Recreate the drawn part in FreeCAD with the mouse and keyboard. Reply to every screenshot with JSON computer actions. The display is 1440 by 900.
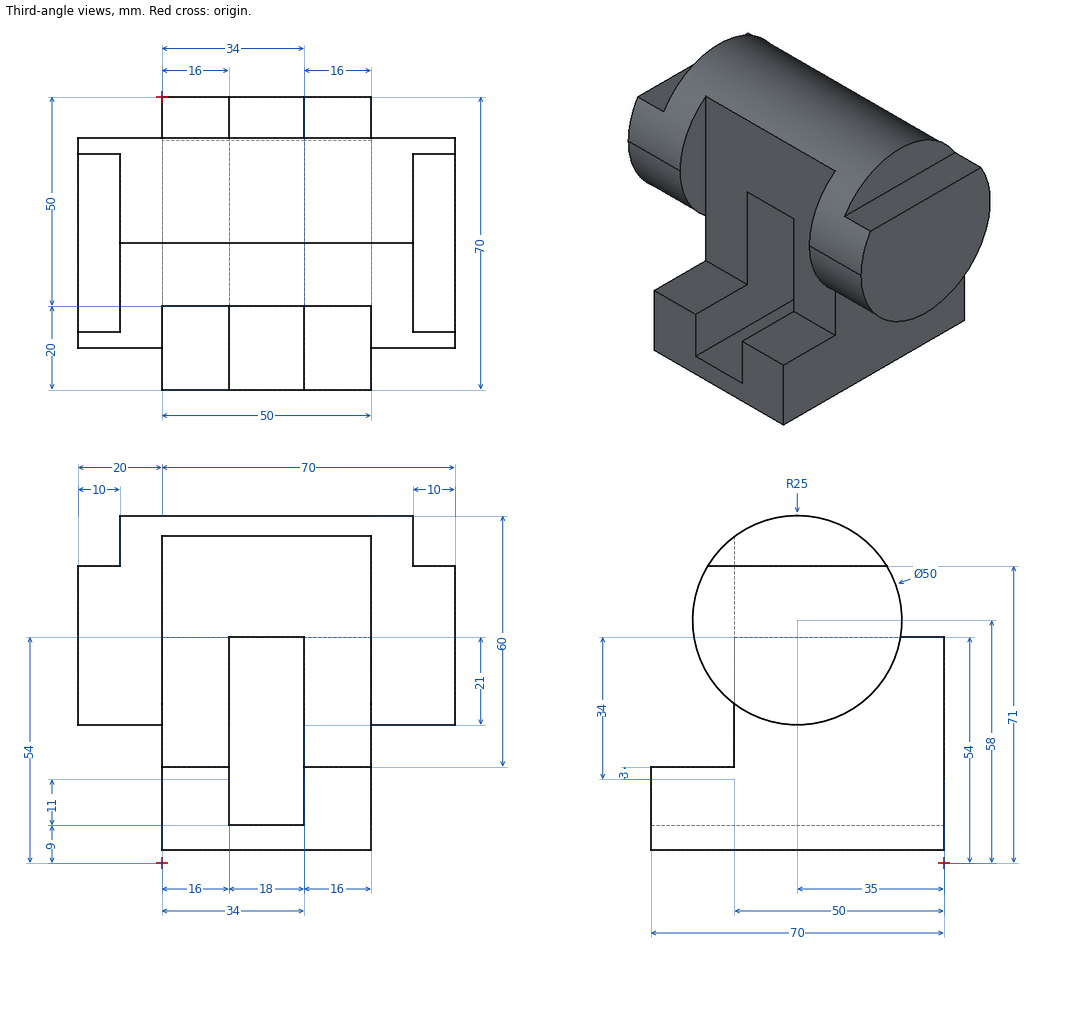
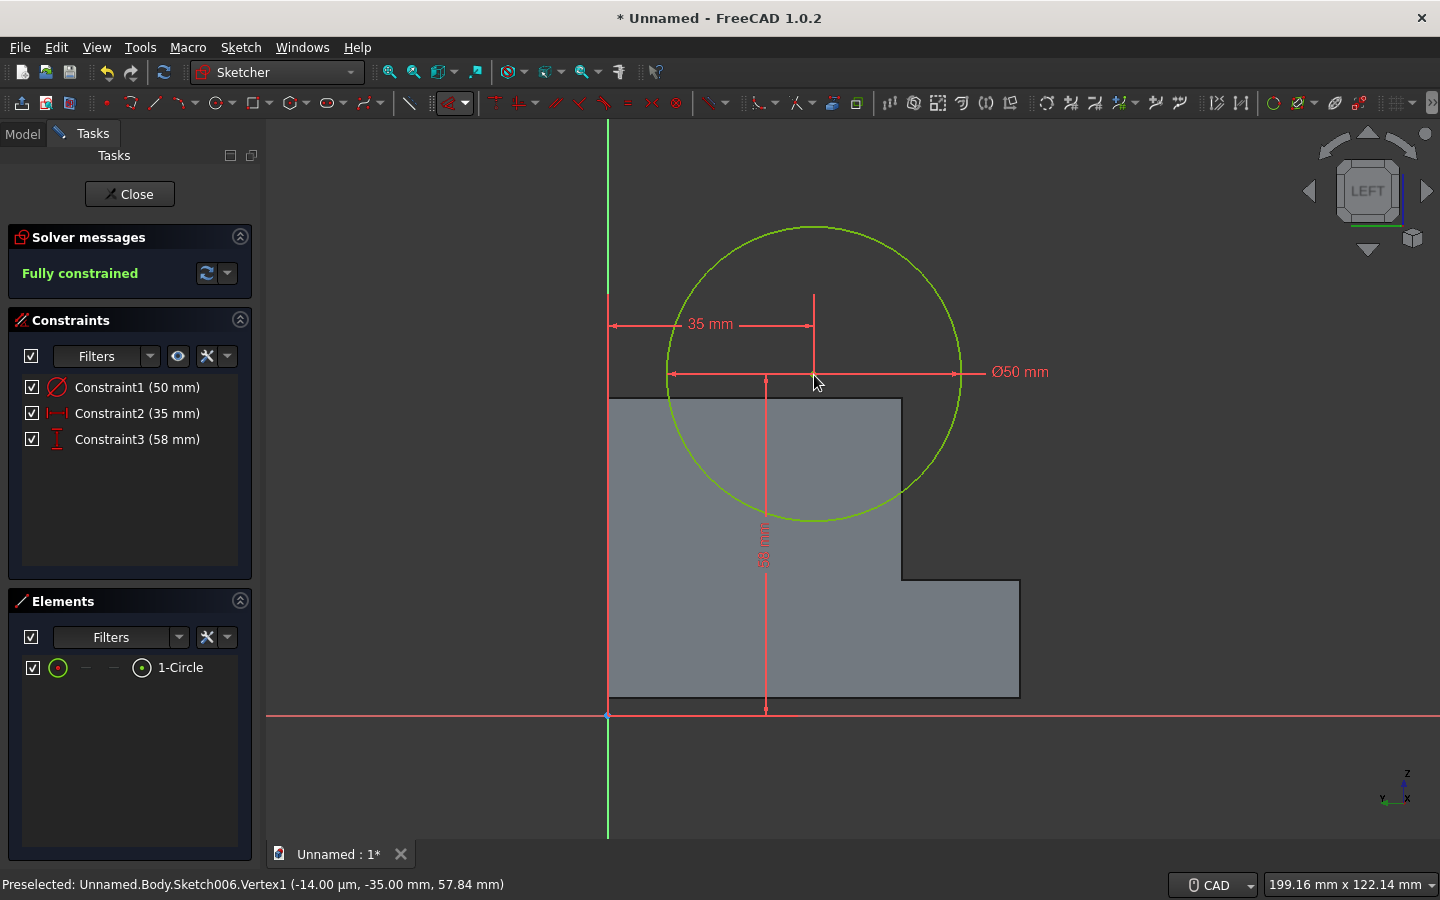
{"action": "left_click", "coordinate": [130, 194]}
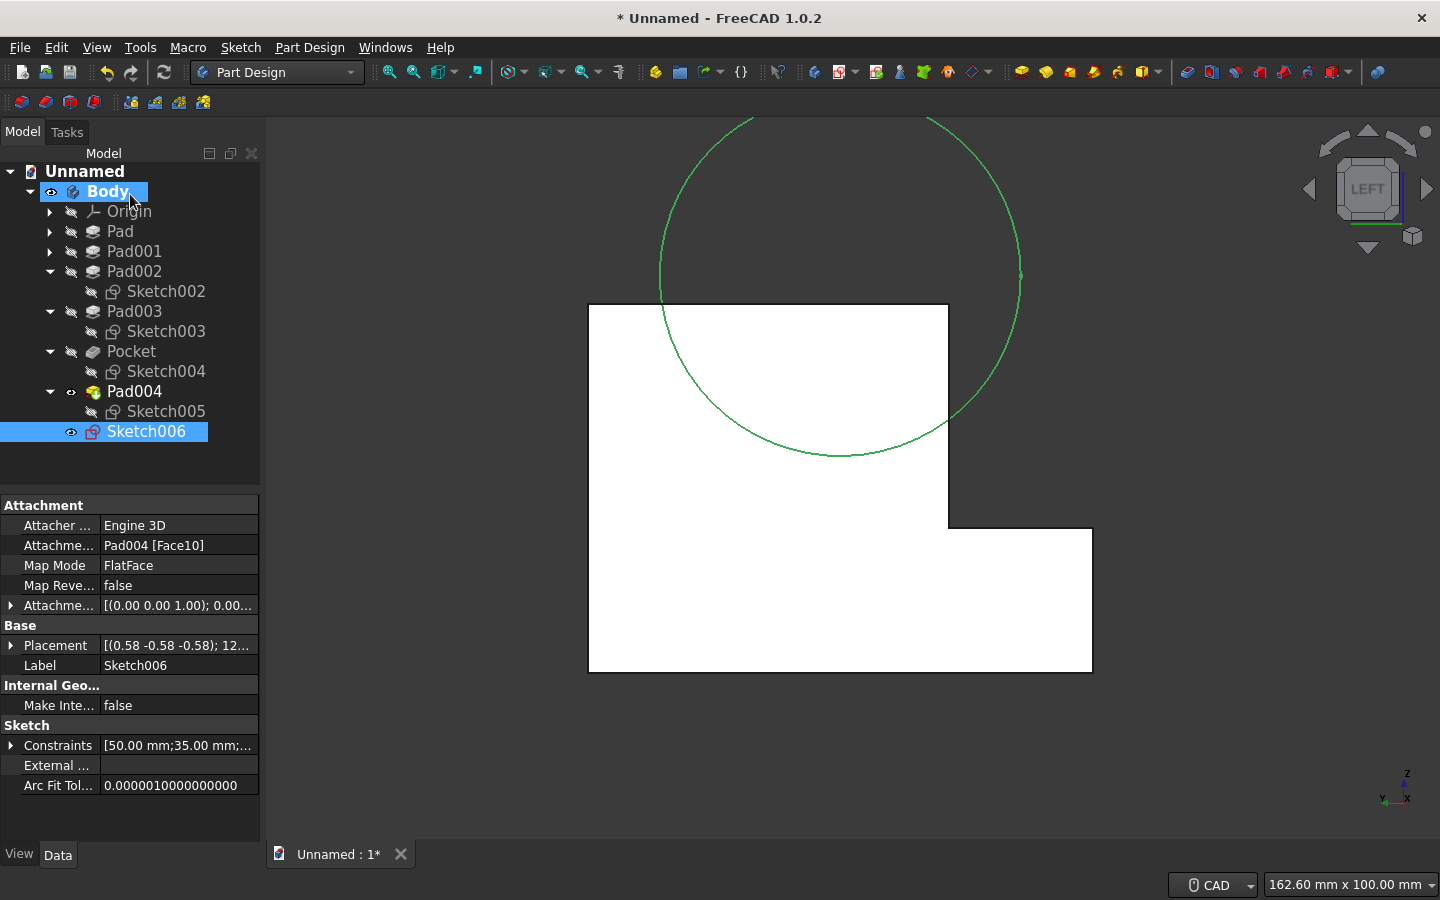
{"action": "left_click", "coordinate": [1022, 72]}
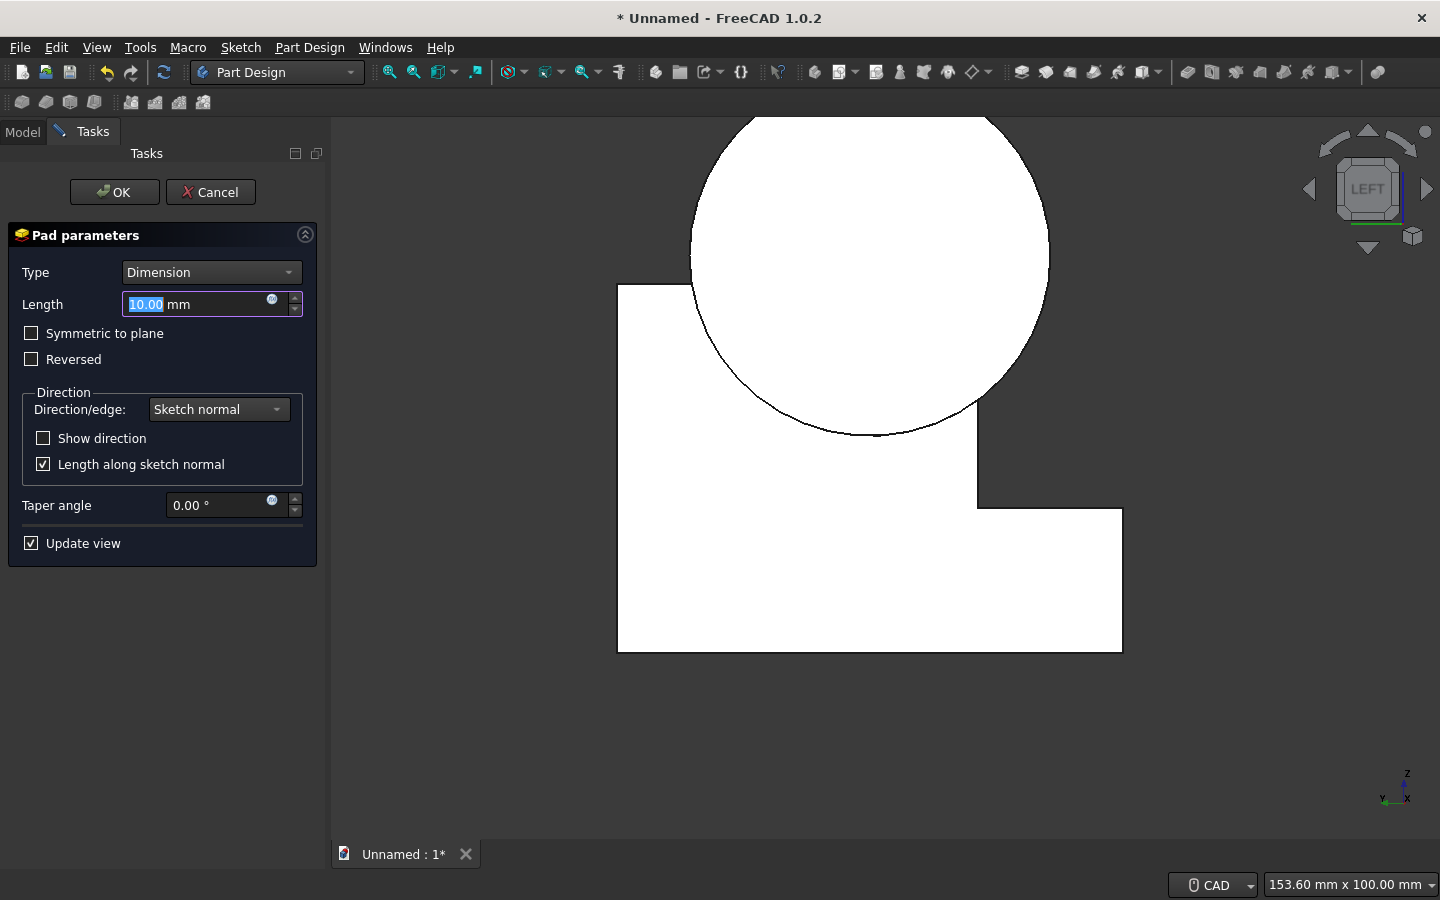
{"action": "type", "text": "70"}
{"action": "key", "text": "Tab"}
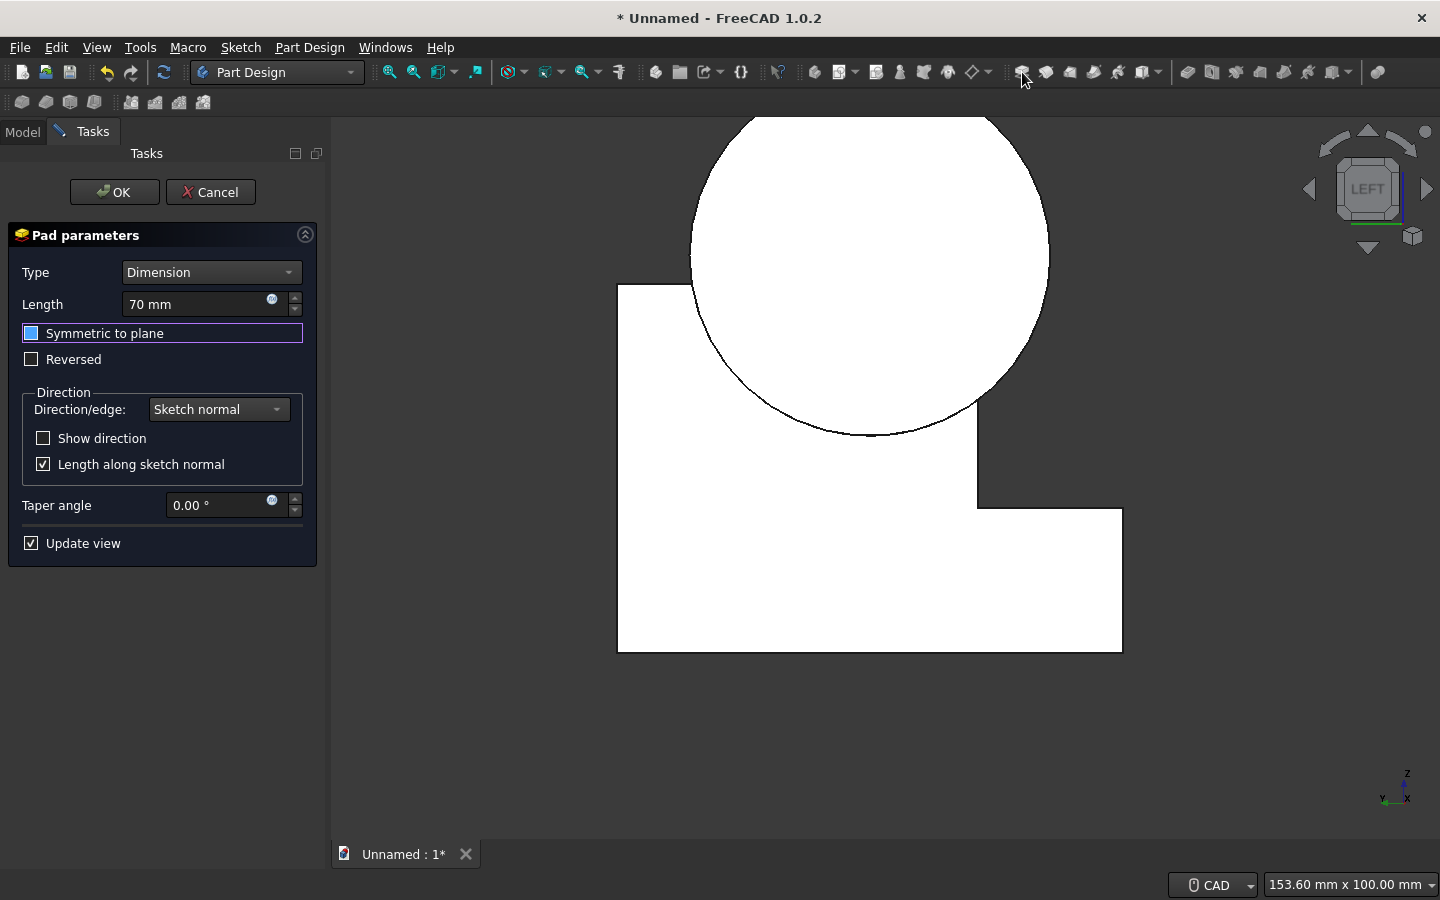
{"action": "left_click", "coordinate": [30, 359]}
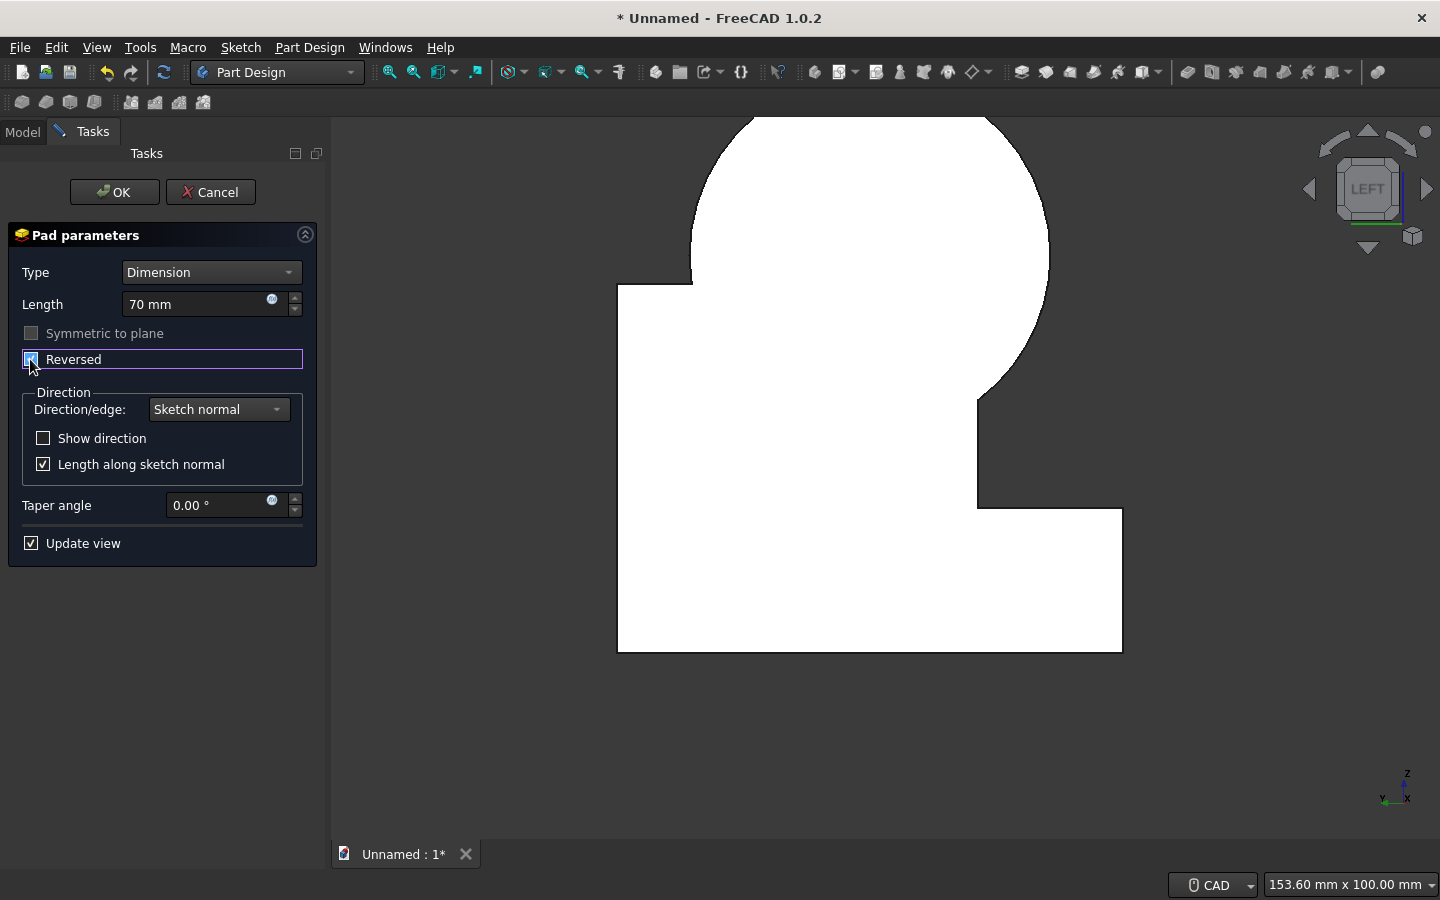
{"action": "left_click", "coordinate": [115, 192]}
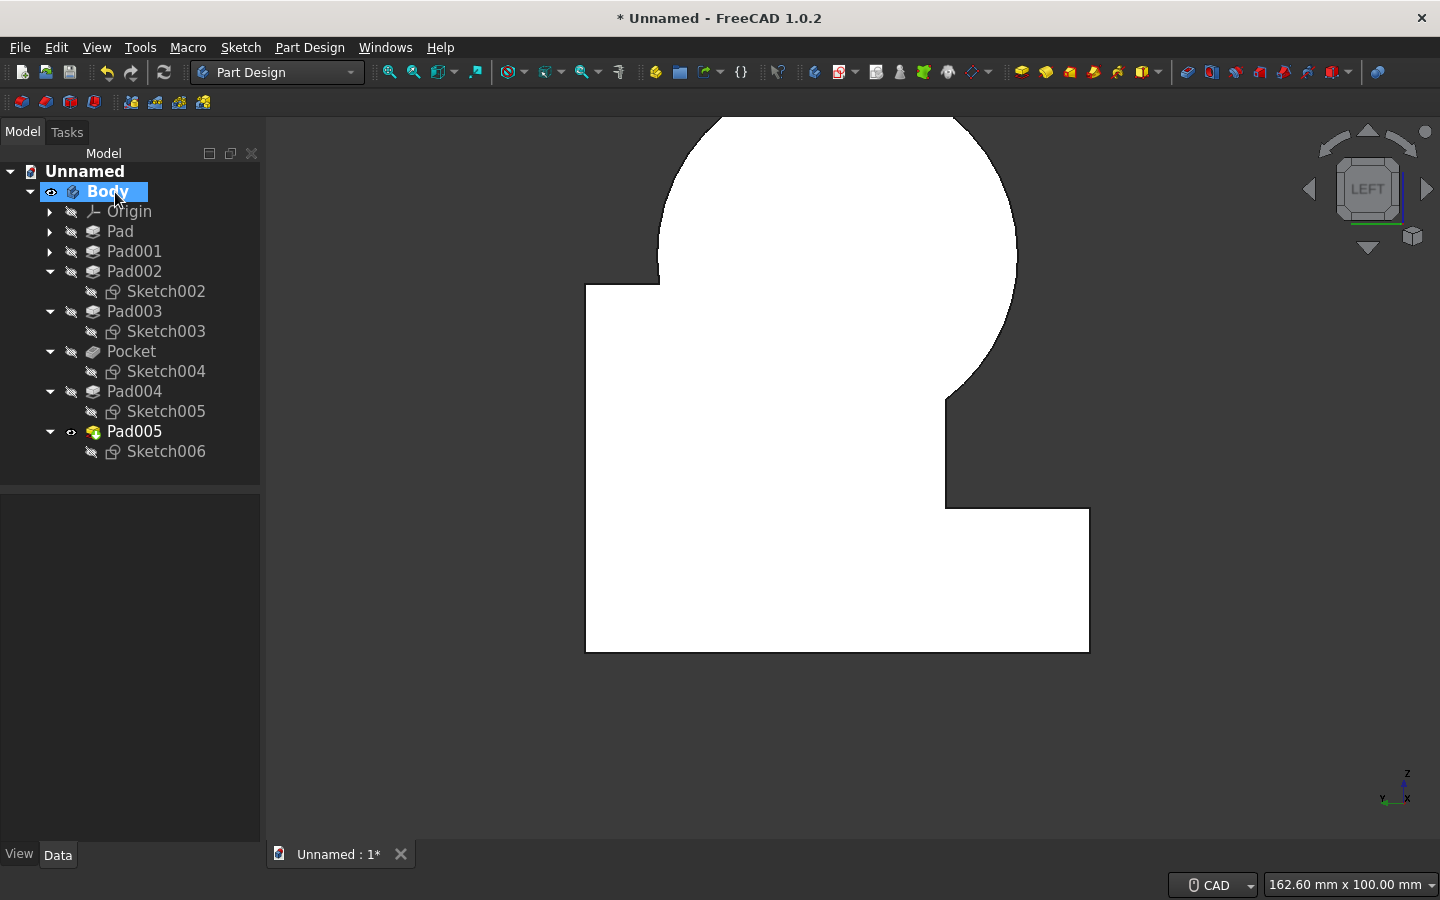
{"action": "key", "text": "v f"}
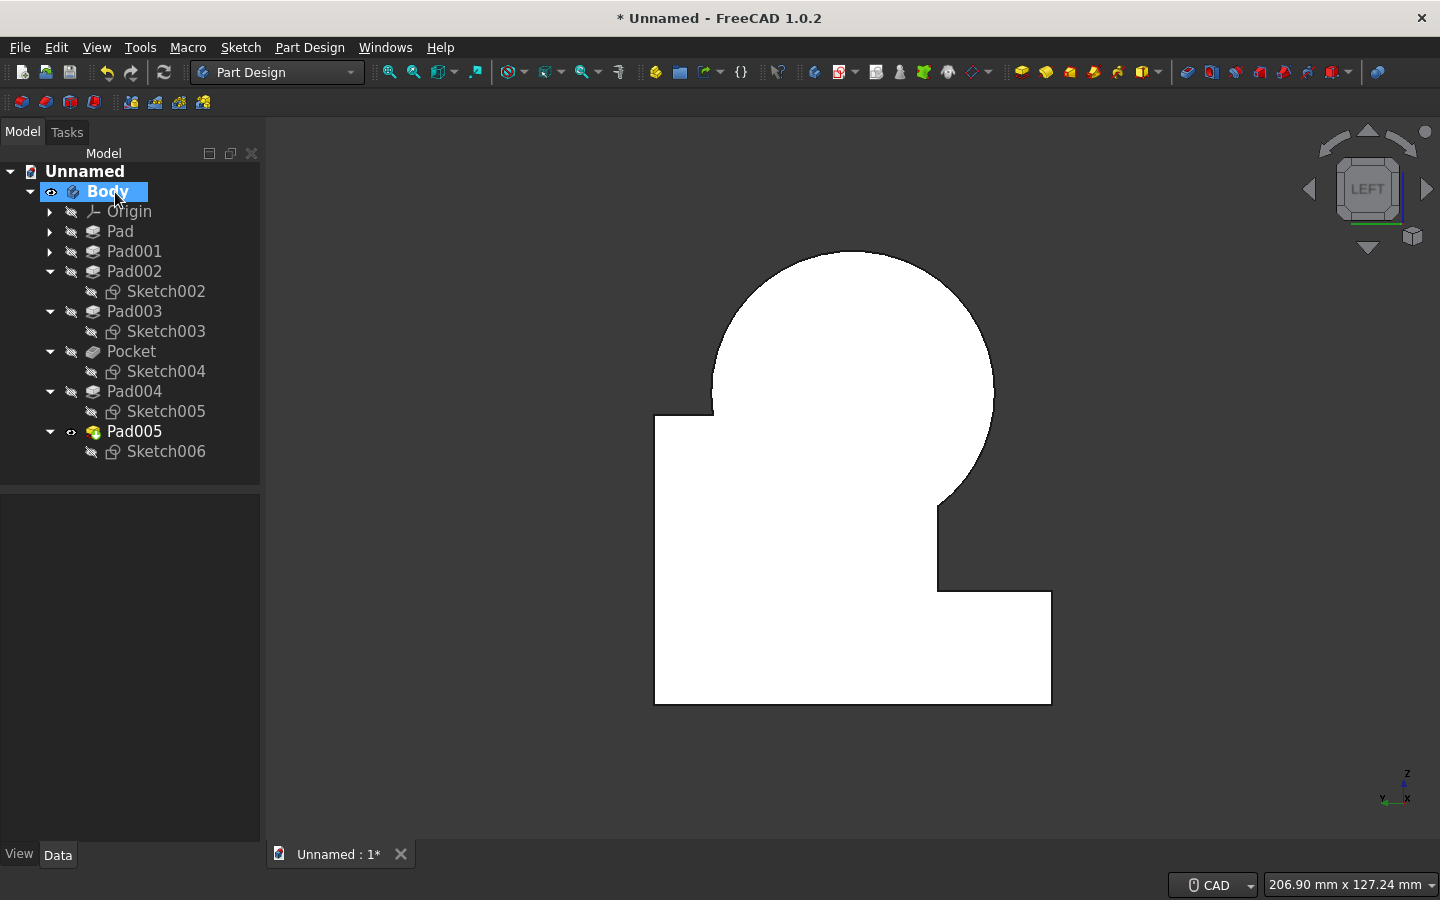
{"action": "left_click", "coordinate": [50, 212]}